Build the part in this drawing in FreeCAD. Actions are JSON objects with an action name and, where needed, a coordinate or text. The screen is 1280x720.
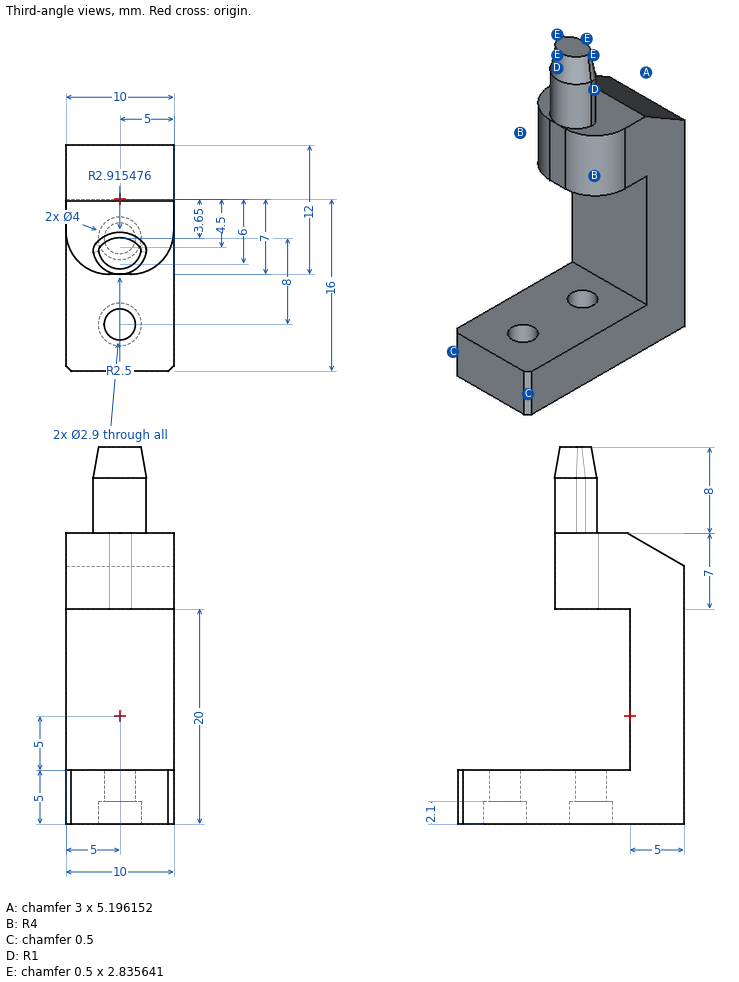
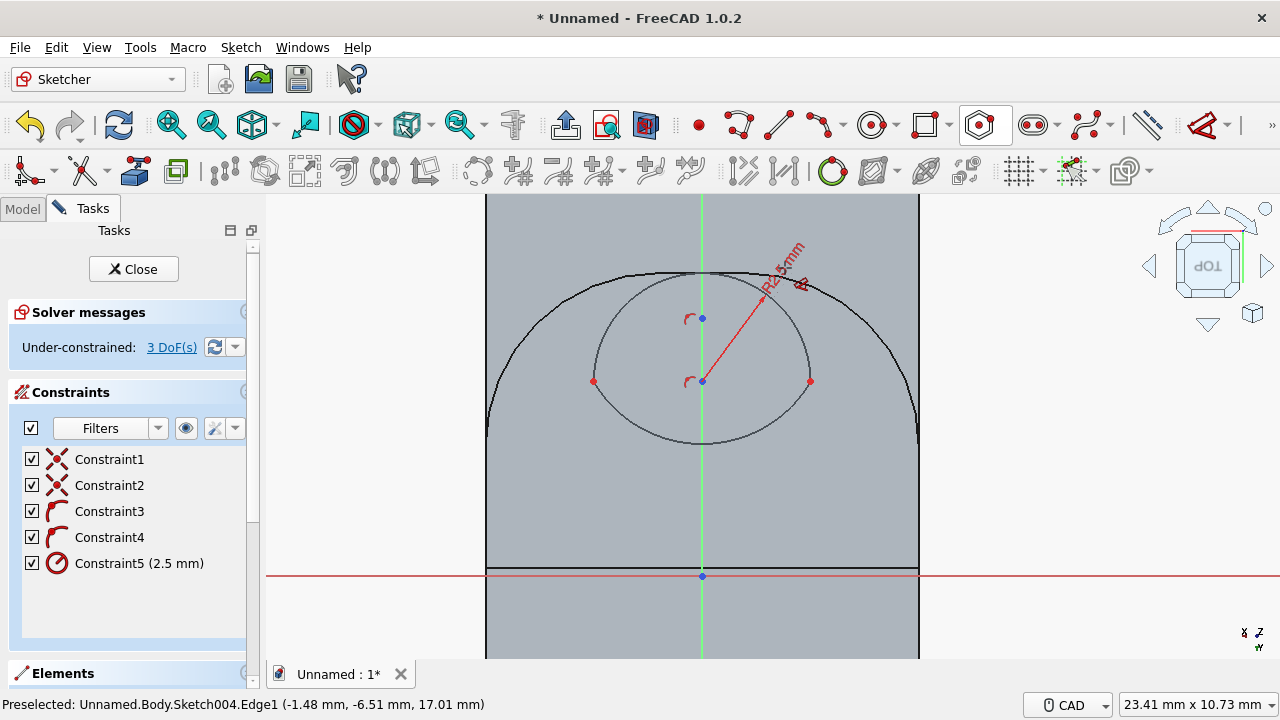
{"action": "left_click", "coordinate": [651, 433]}
{"action": "left_click", "coordinate": [638, 462]}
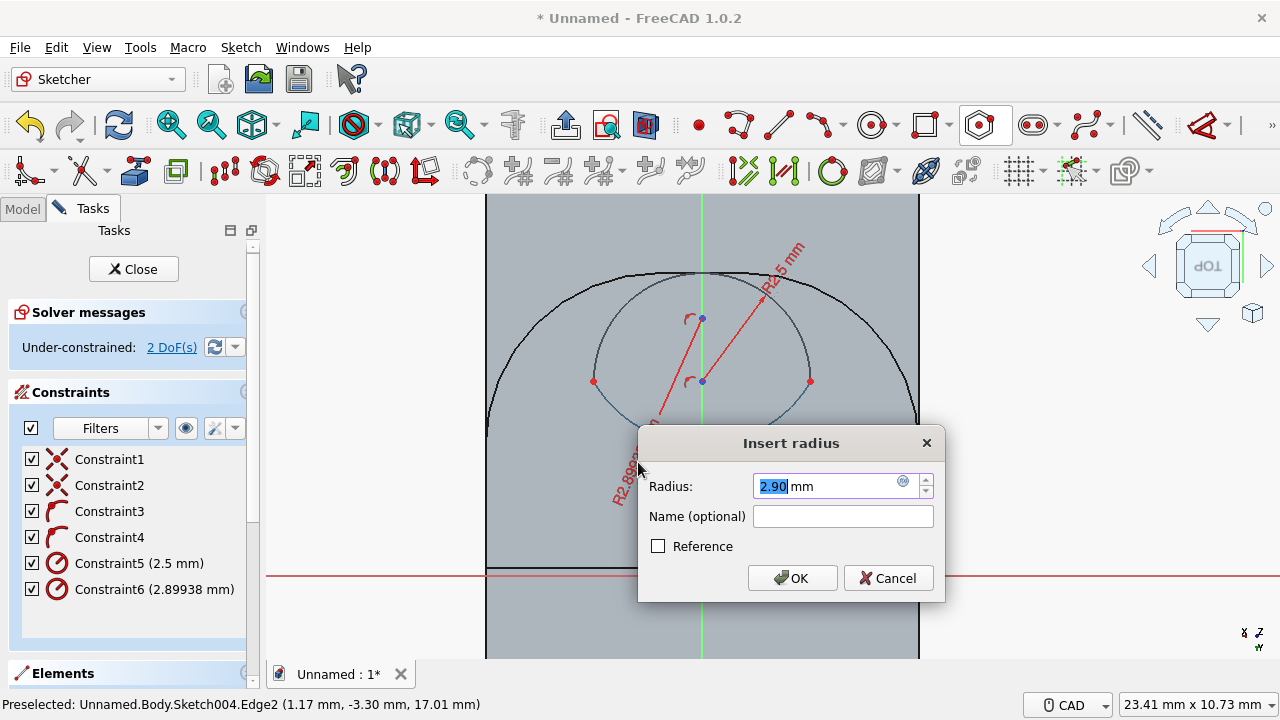
{"action": "type", "text": "2.915476"}
{"action": "key", "text": "Return"}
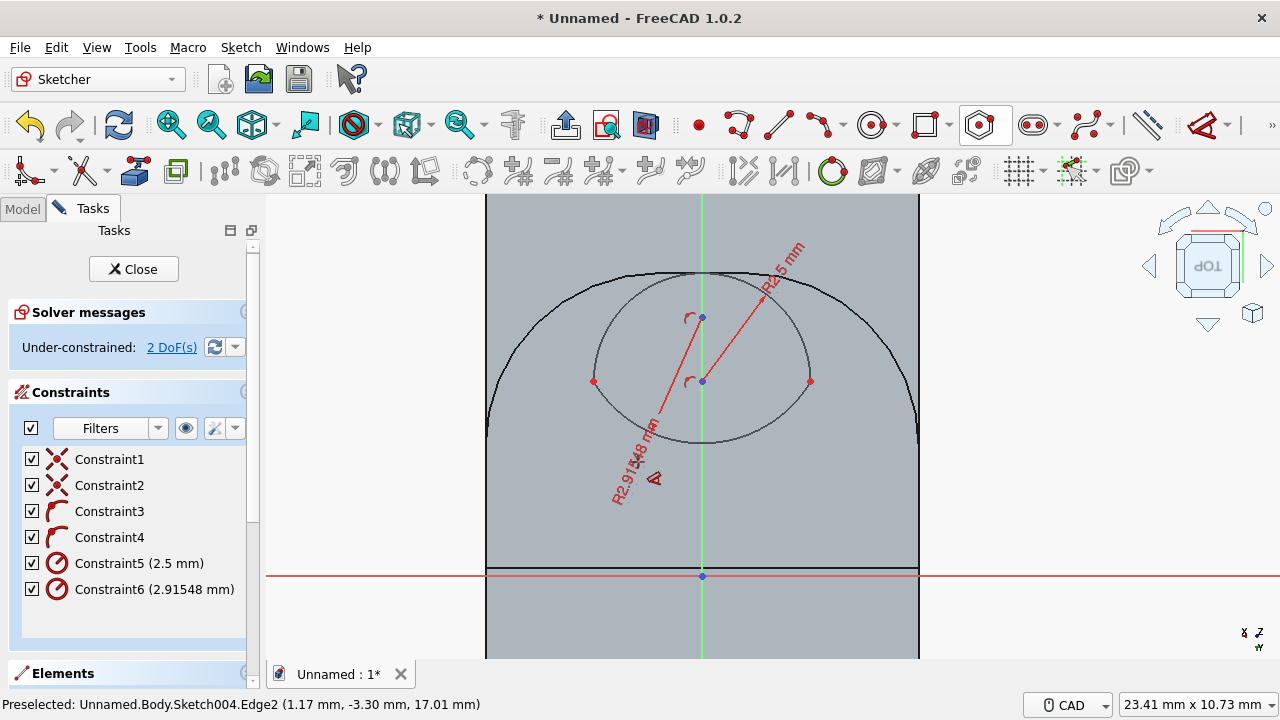
{"action": "left_click", "coordinate": [702, 317]}
{"action": "left_click", "coordinate": [736, 387]}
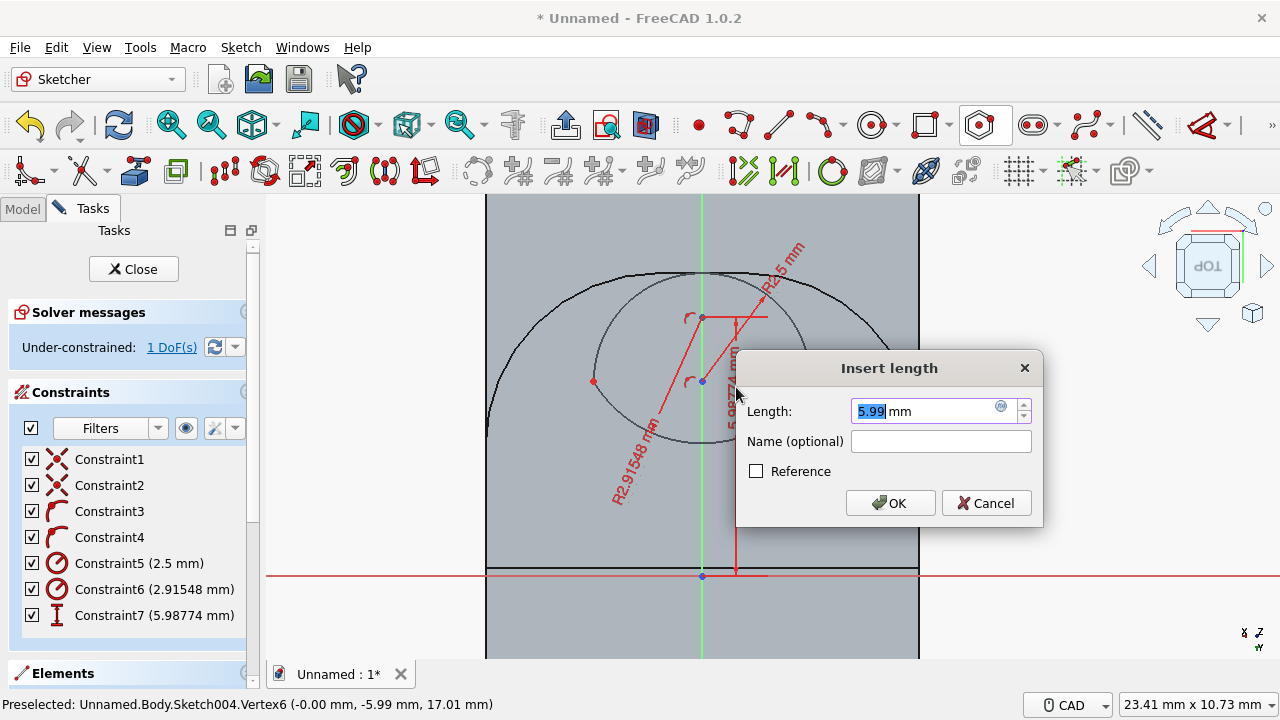
{"action": "type", "text": "6"}
{"action": "key", "text": "Return"}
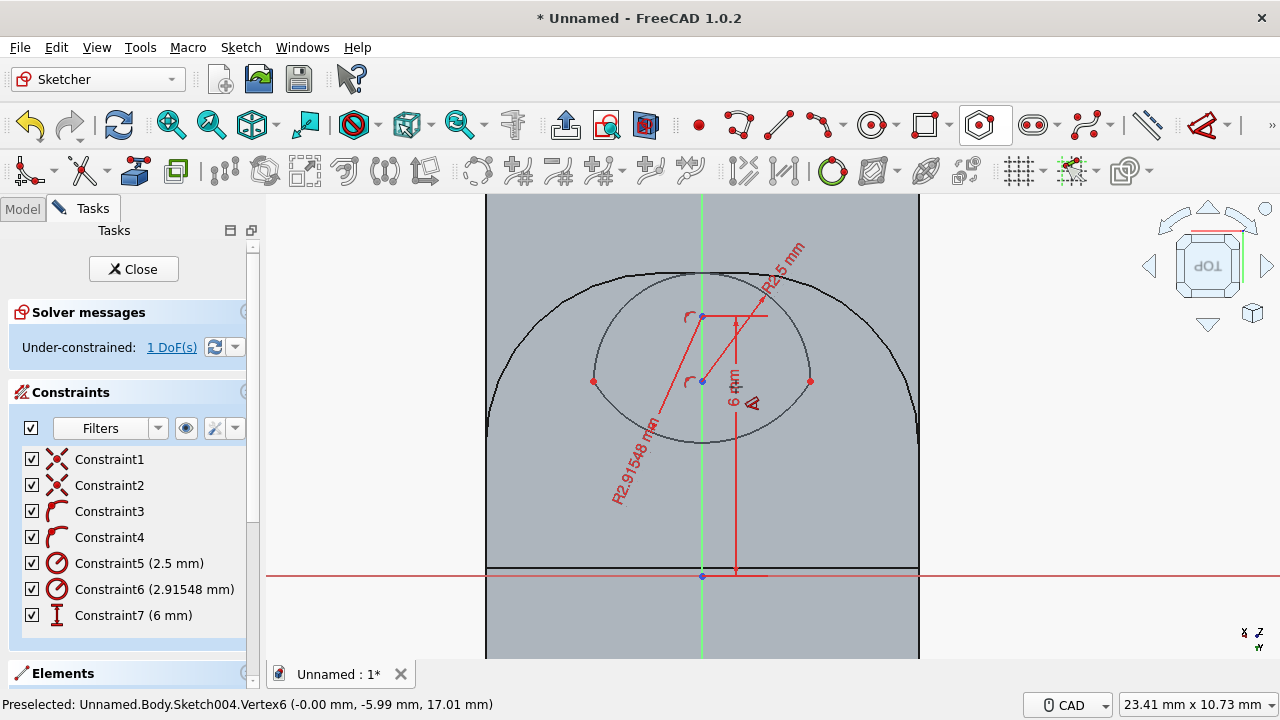
{"action": "left_click", "coordinate": [702, 382]}
{"action": "left_click", "coordinate": [736, 479]}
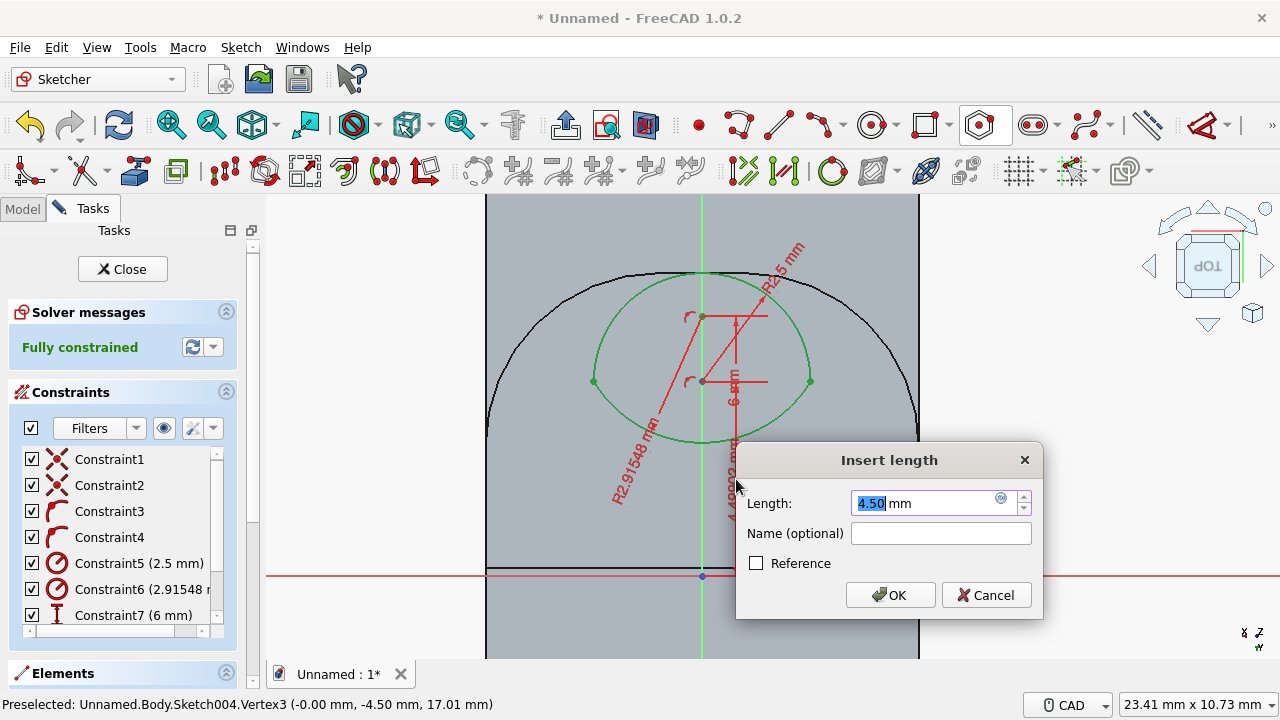
{"action": "type", "text": "4.5"}
{"action": "key", "text": "Return"}
{"action": "key", "text": "Escape"}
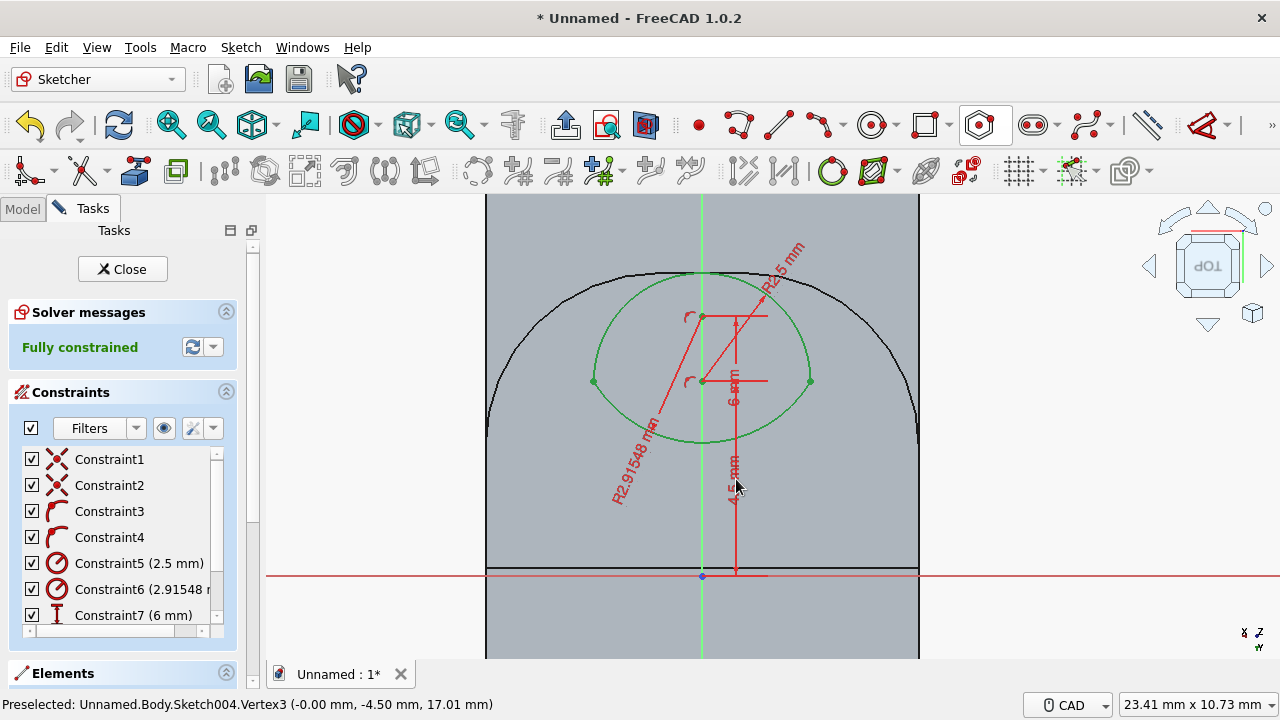
{"action": "left_click", "coordinate": [123, 269]}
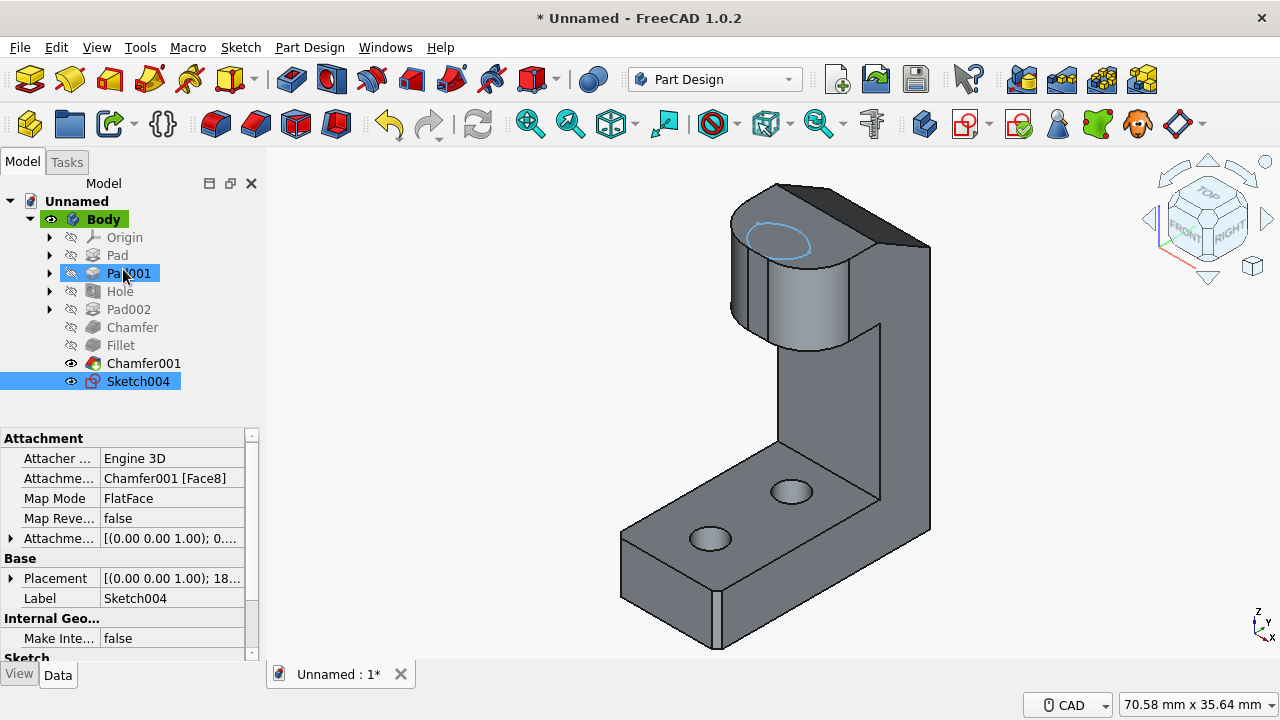
{"action": "left_click", "coordinate": [30, 80]}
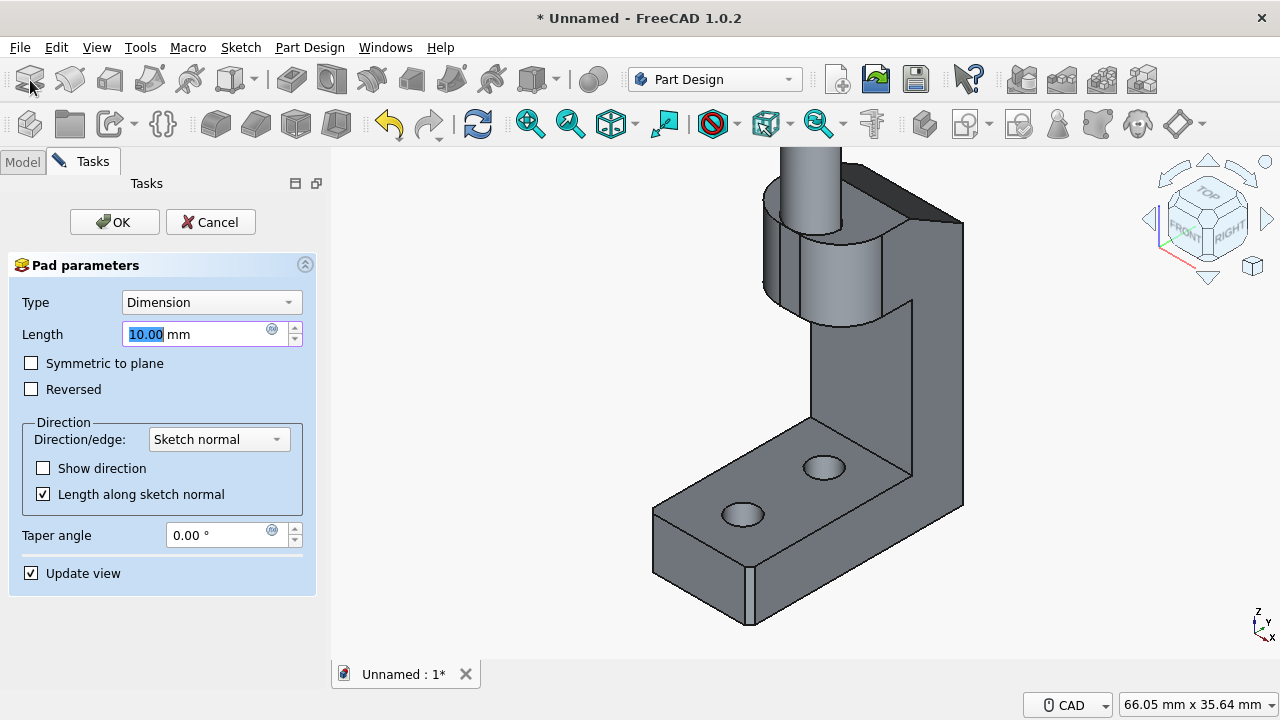
{"action": "type", "text": "8"}
{"action": "key", "text": "Tab"}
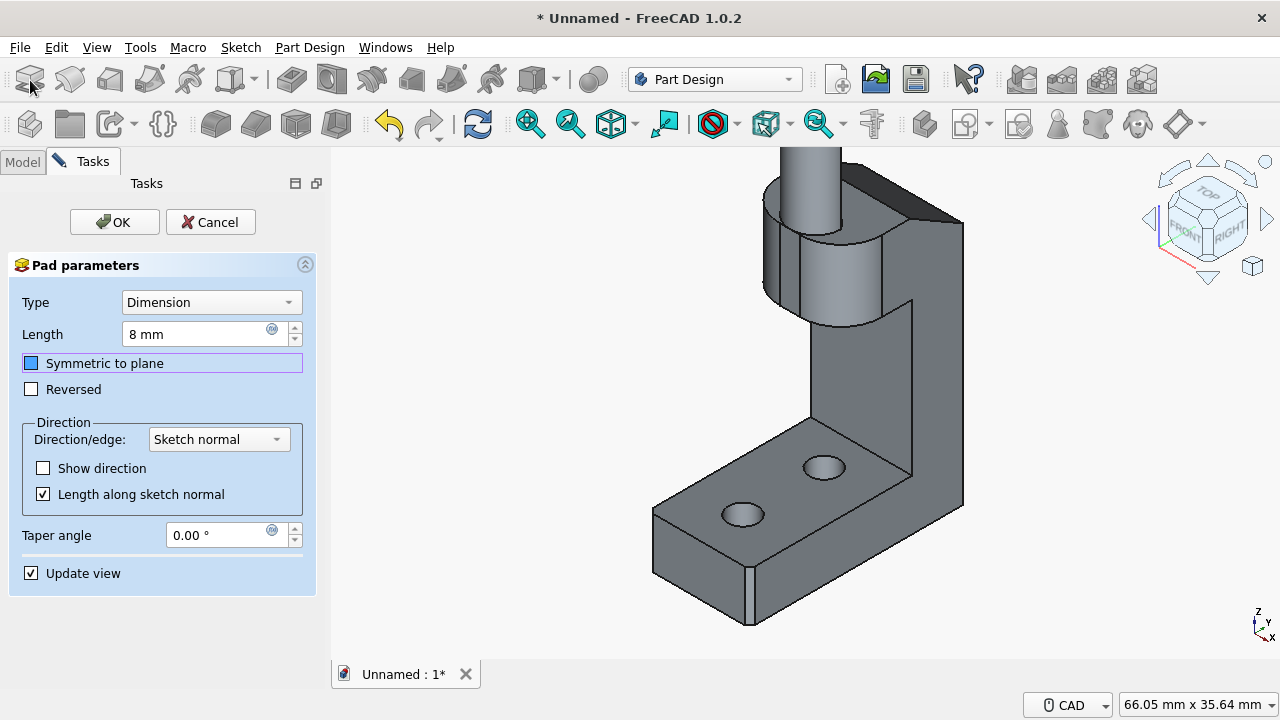
{"action": "left_click", "coordinate": [115, 222]}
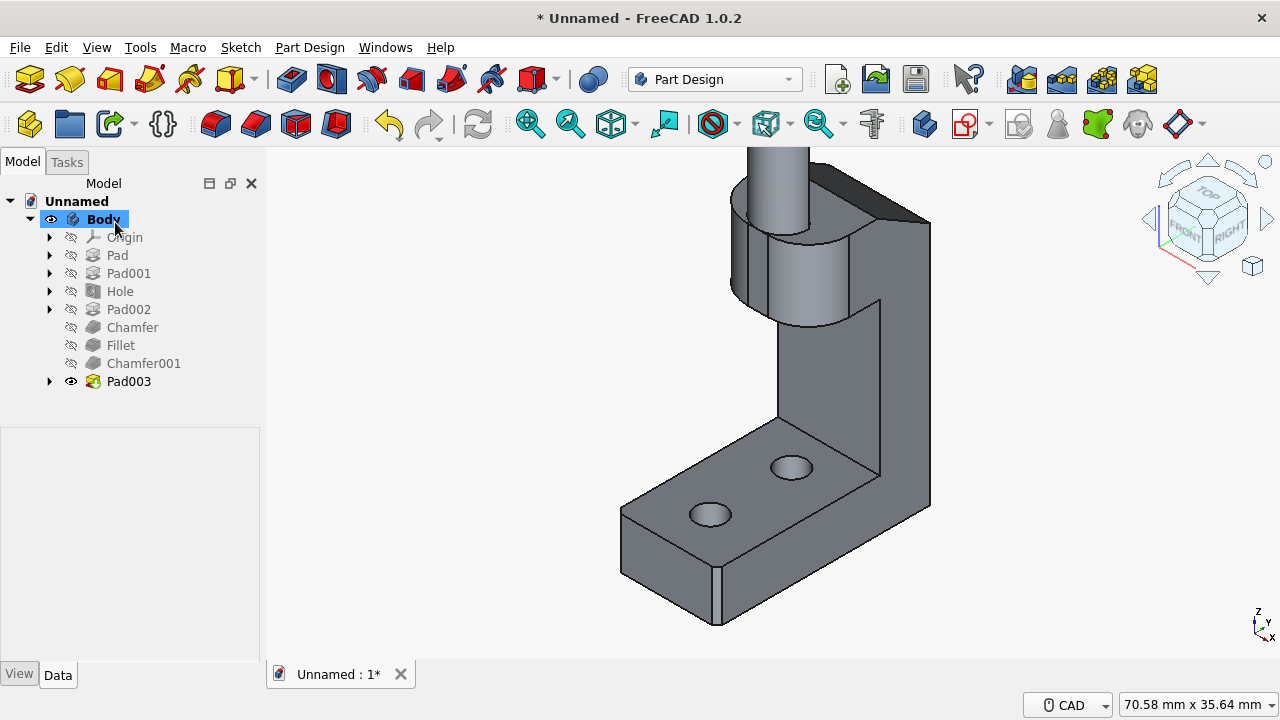
{"action": "left_click", "coordinate": [532, 124]}